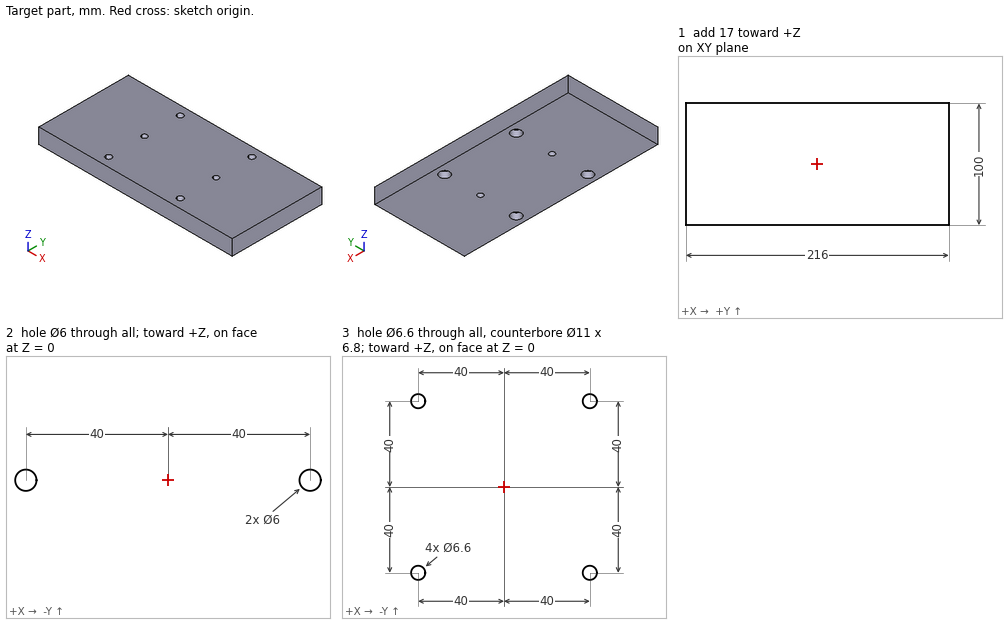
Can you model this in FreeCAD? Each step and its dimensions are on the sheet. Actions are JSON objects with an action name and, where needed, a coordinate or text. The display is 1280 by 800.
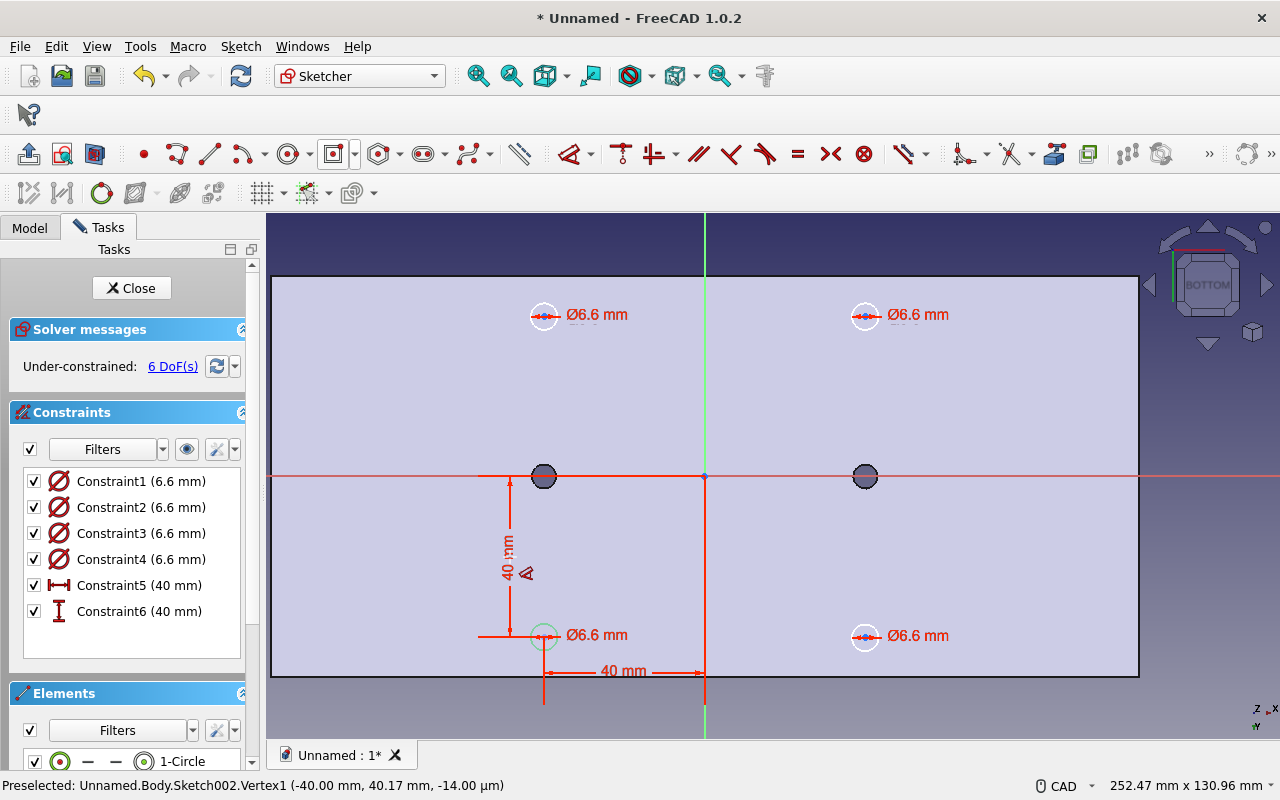
{"action": "left_click", "coordinate": [544, 317]}
{"action": "left_click", "coordinate": [624, 283]}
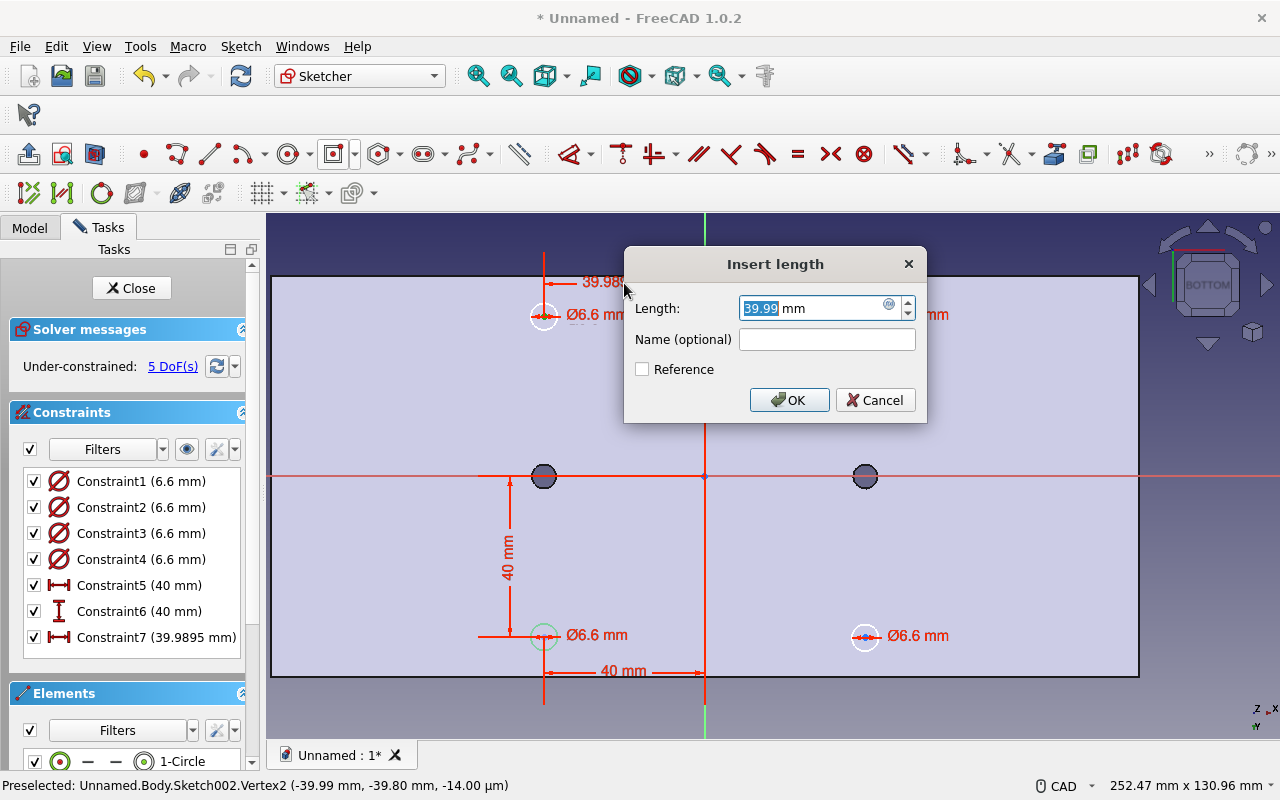
{"action": "type", "text": "40"}
{"action": "key", "text": "Return"}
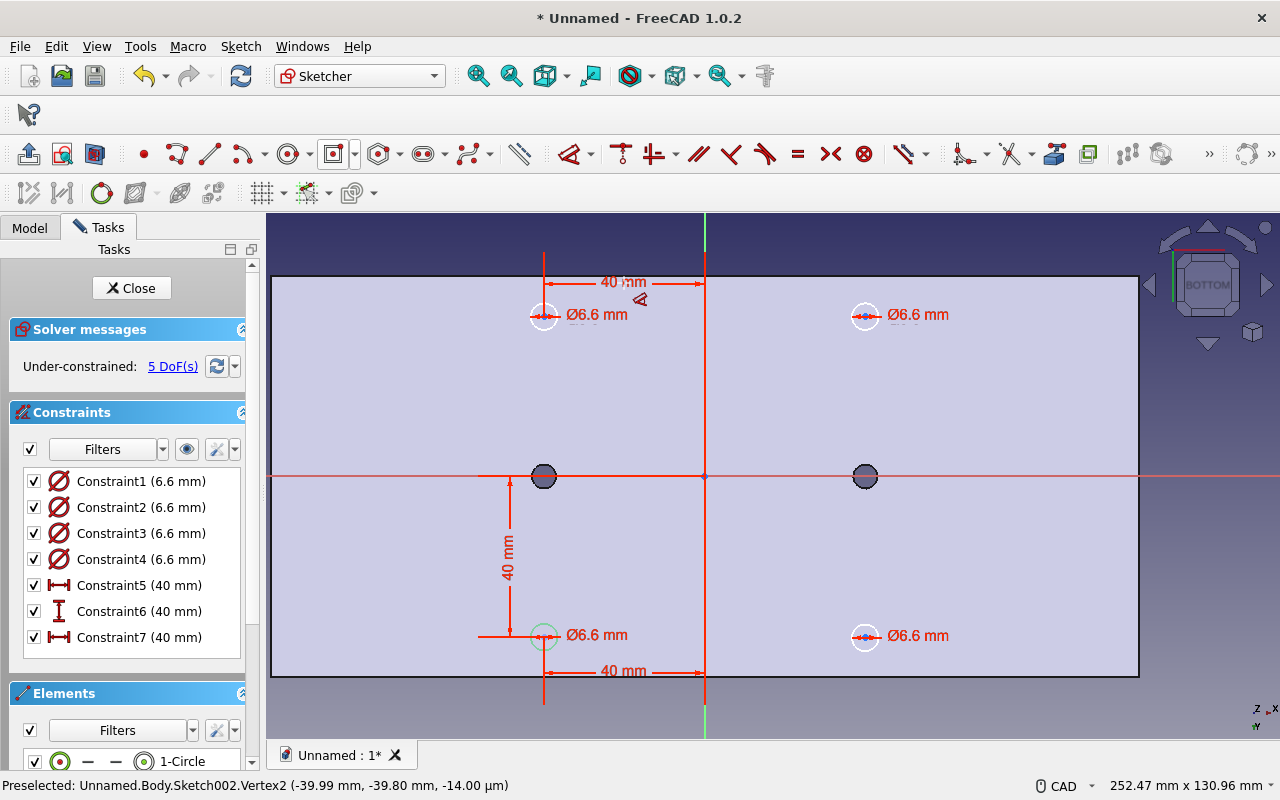
{"action": "left_click", "coordinate": [544, 317]}
{"action": "left_click", "coordinate": [510, 397]}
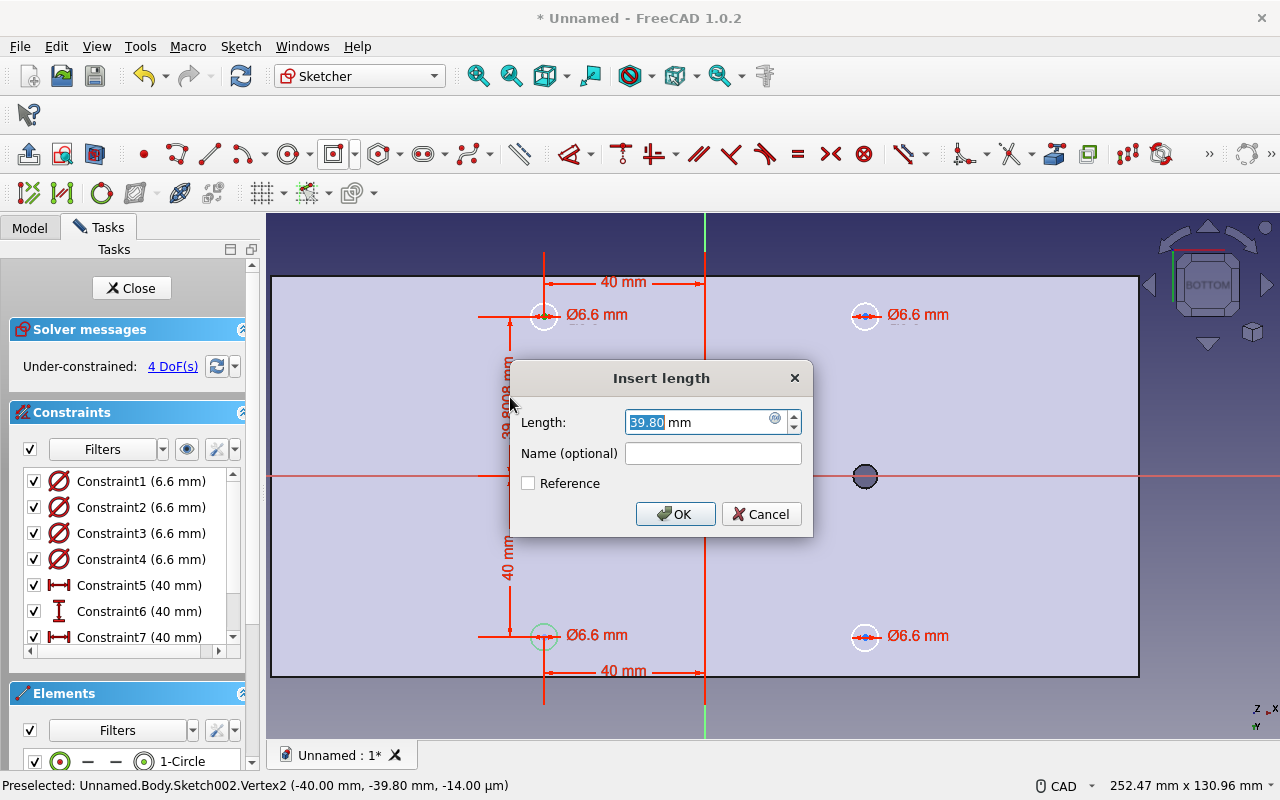
{"action": "type", "text": "40"}
{"action": "key", "text": "Return"}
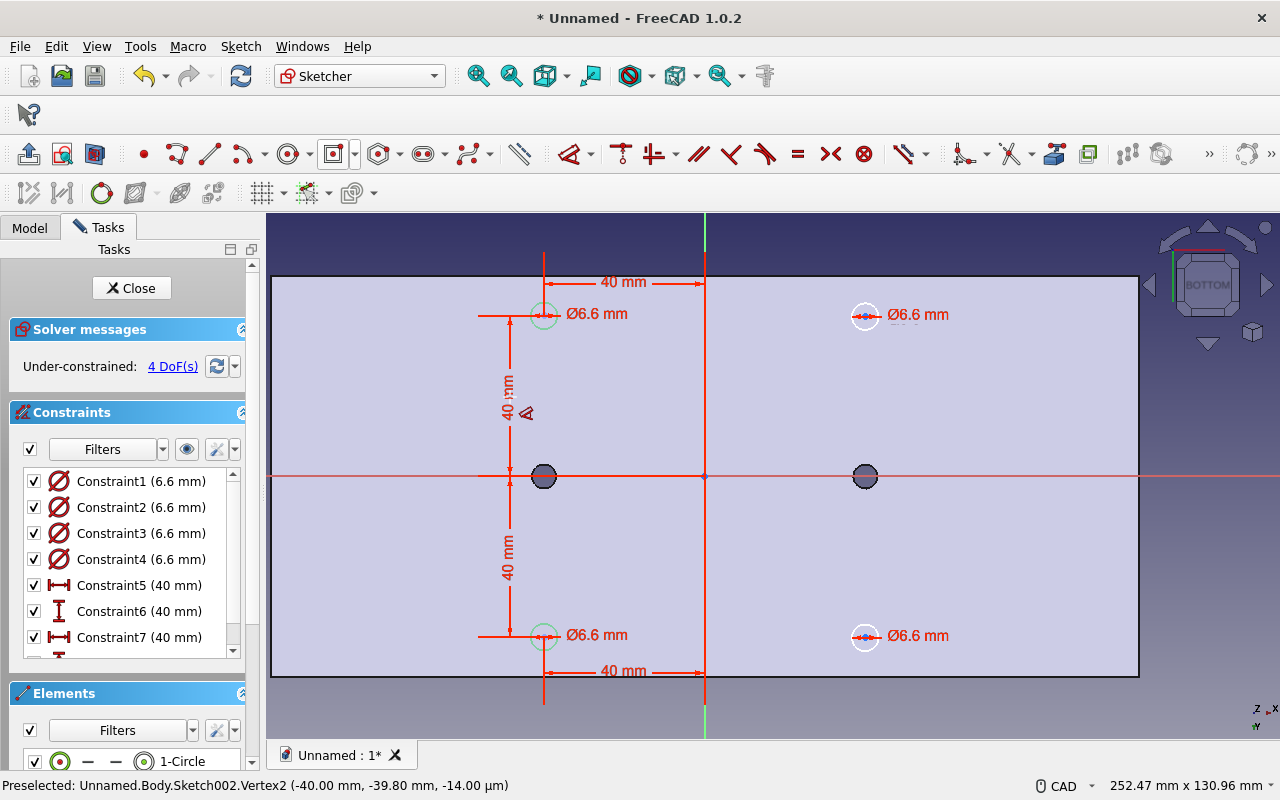
{"action": "left_click", "coordinate": [865, 317]}
{"action": "left_click", "coordinate": [785, 283]}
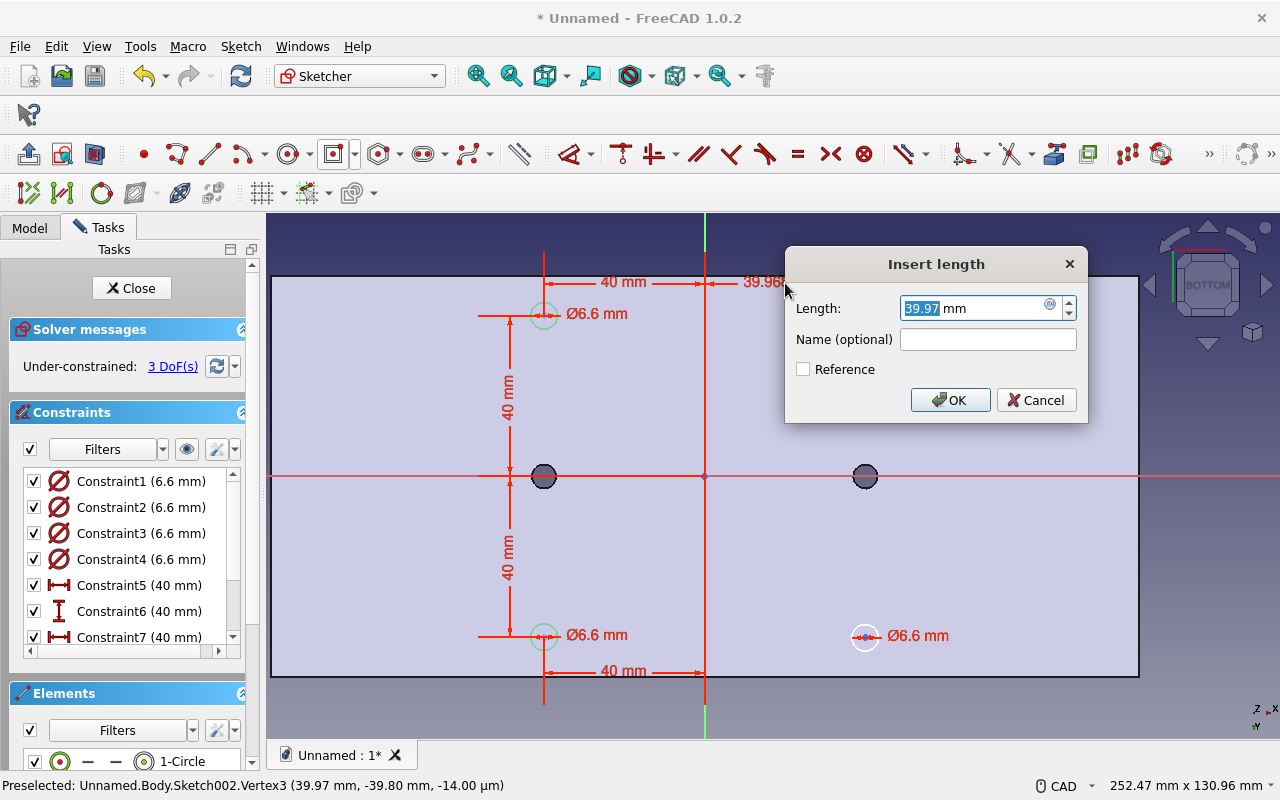
{"action": "type", "text": "40"}
{"action": "key", "text": "Return"}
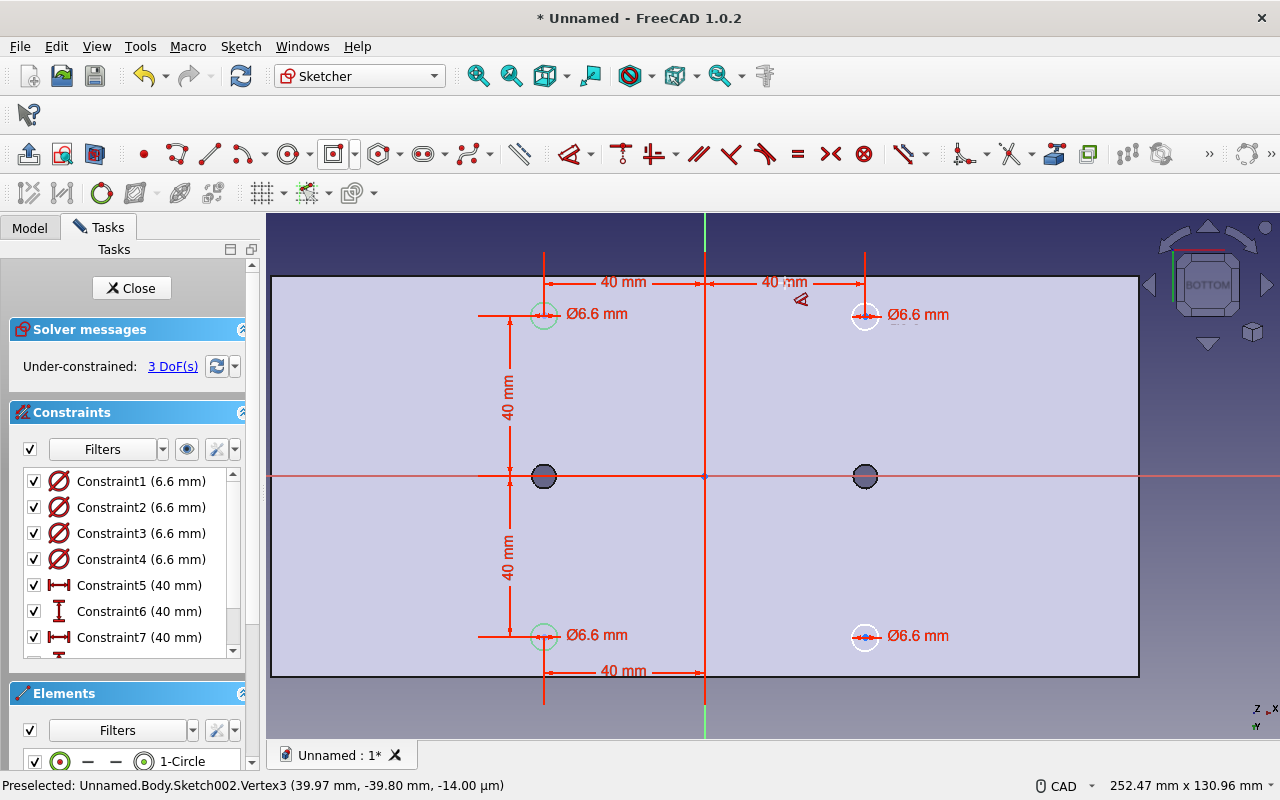
{"action": "left_click", "coordinate": [865, 317]}
{"action": "left_click", "coordinate": [899, 397]}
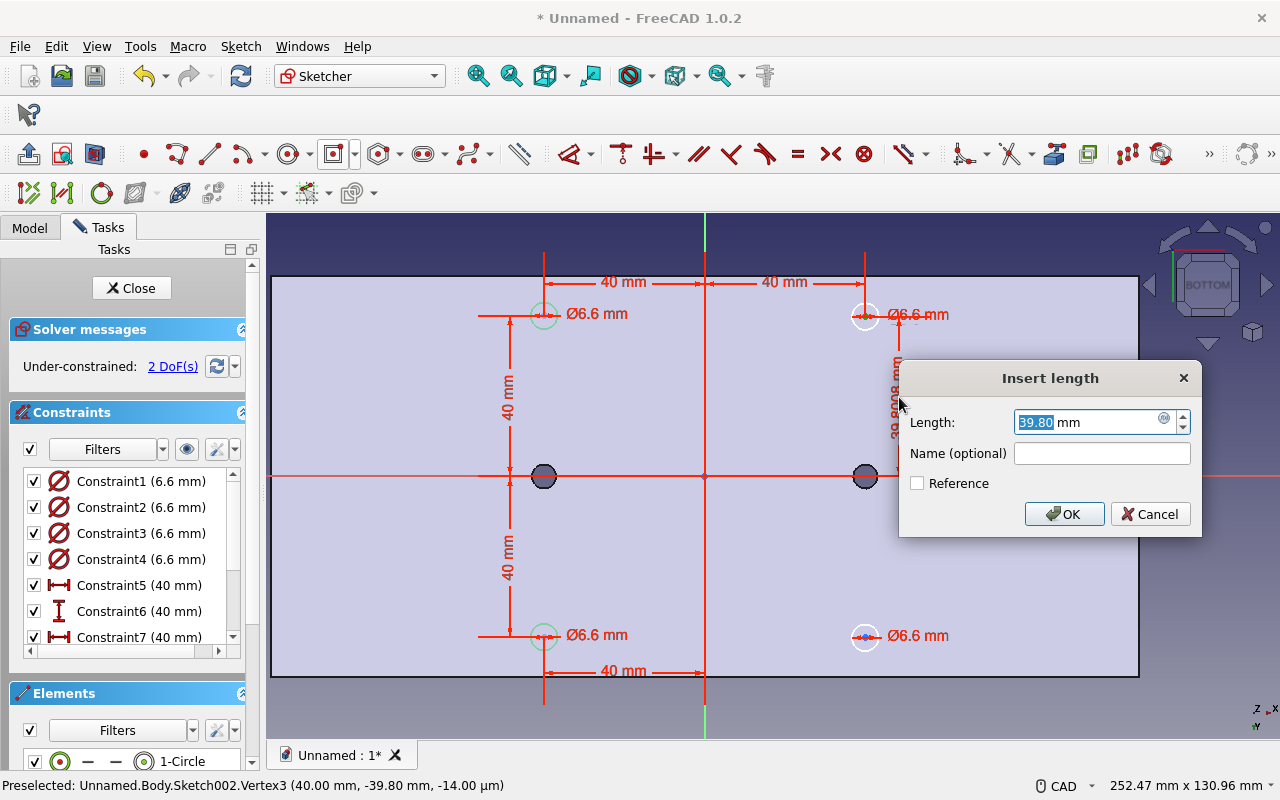
{"action": "type", "text": "40"}
{"action": "key", "text": "Return"}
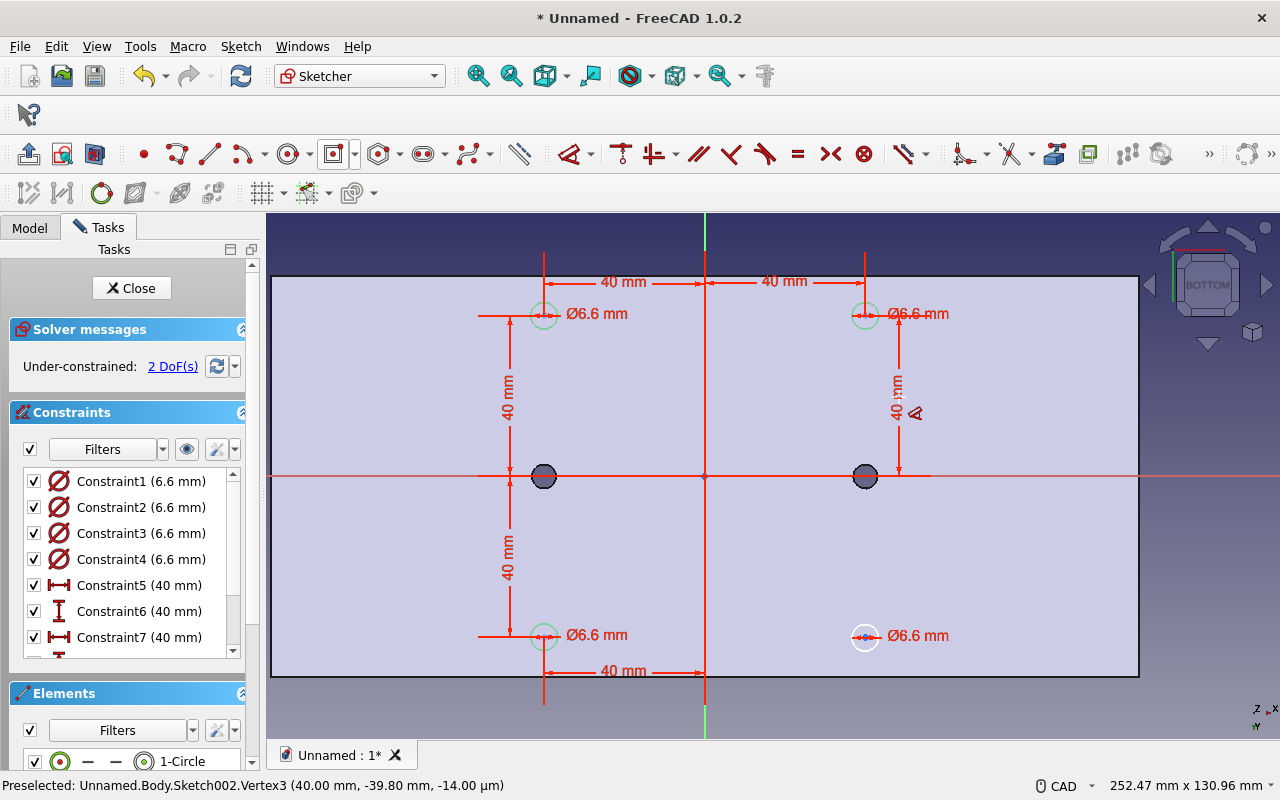
{"action": "left_click", "coordinate": [865, 638]}
{"action": "left_click", "coordinate": [785, 672]}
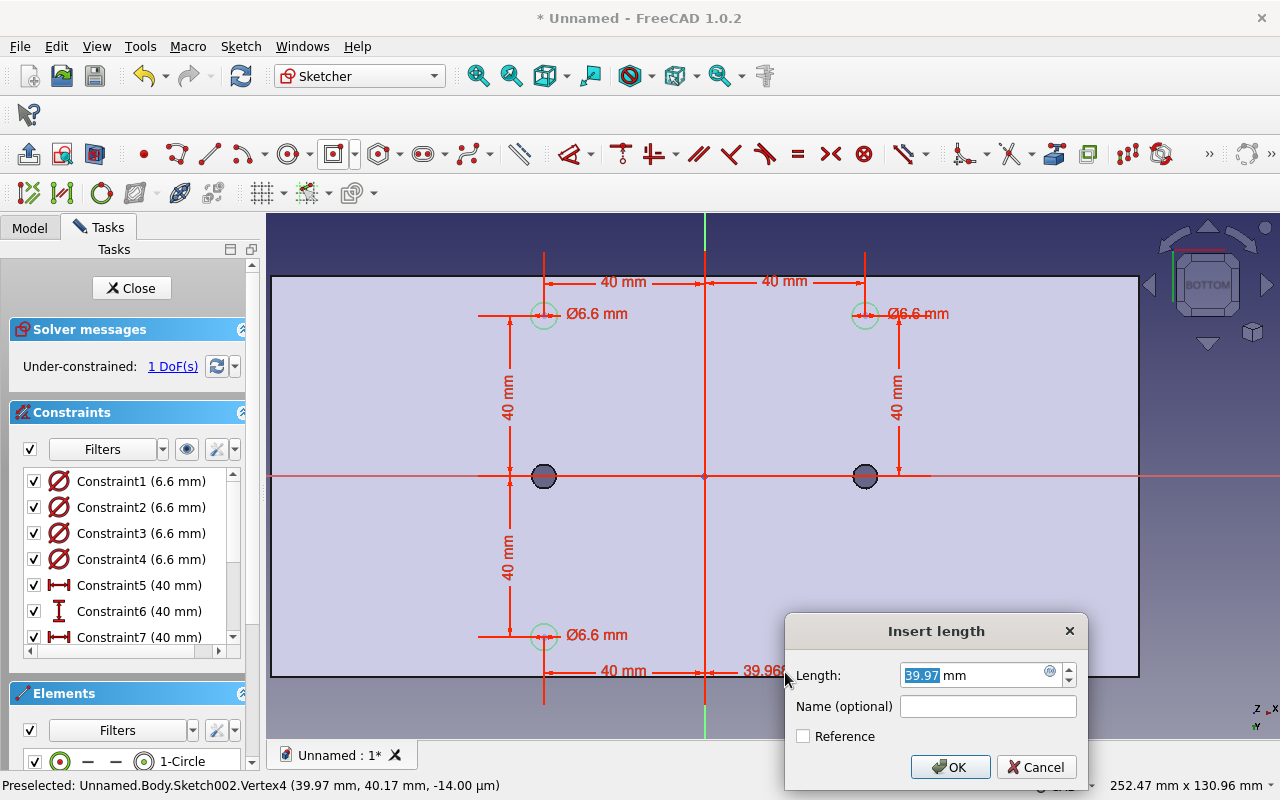
{"action": "type", "text": "40"}
{"action": "key", "text": "Return"}